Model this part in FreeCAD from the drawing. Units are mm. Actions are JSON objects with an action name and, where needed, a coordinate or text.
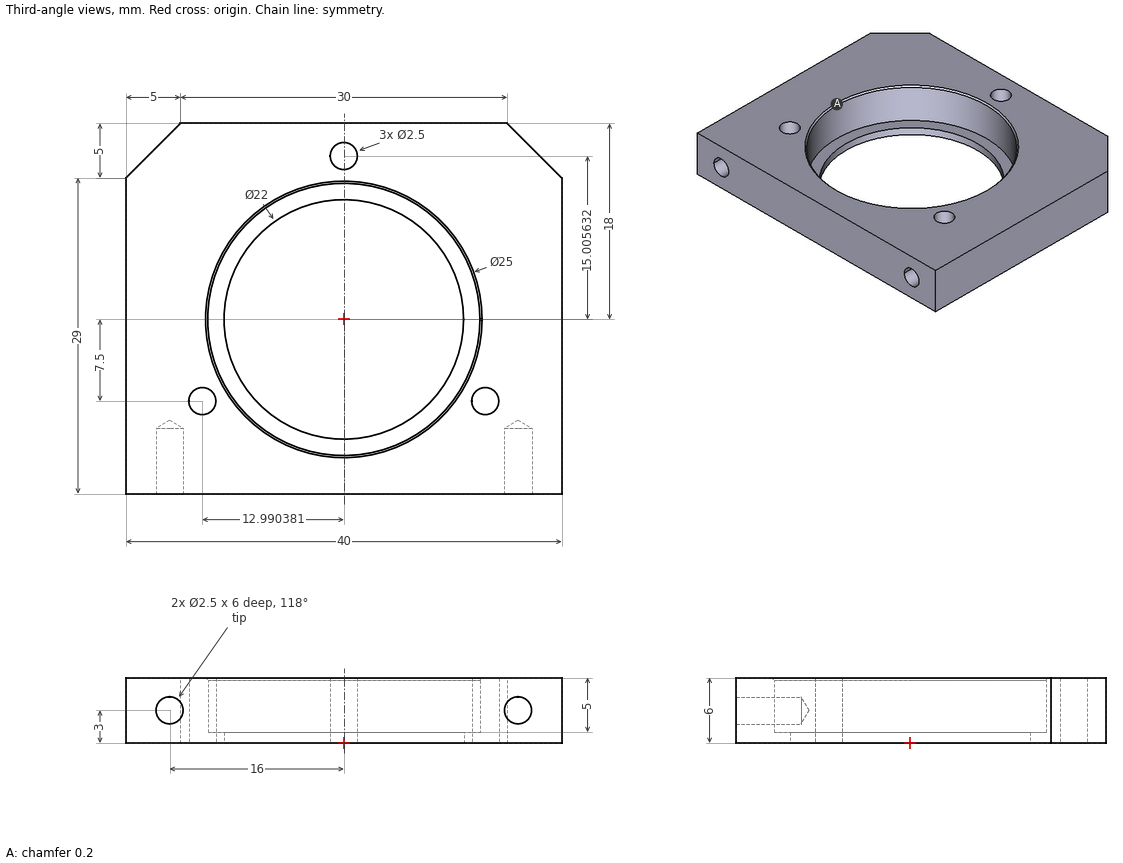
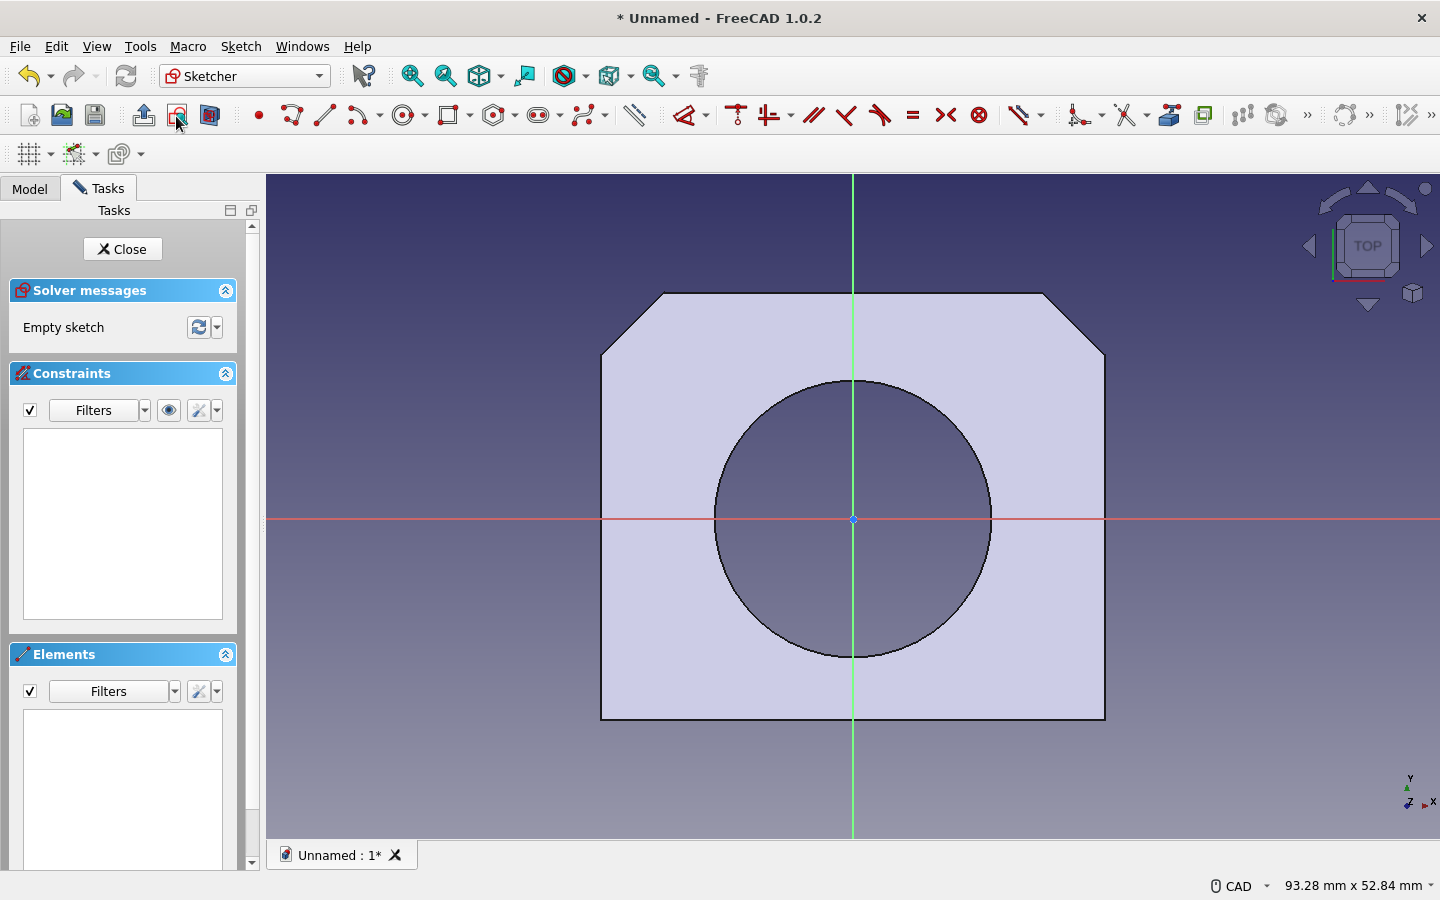
{"action": "scroll", "coordinate": [992, 545], "scroll_direction": "up", "scroll_amount": 2}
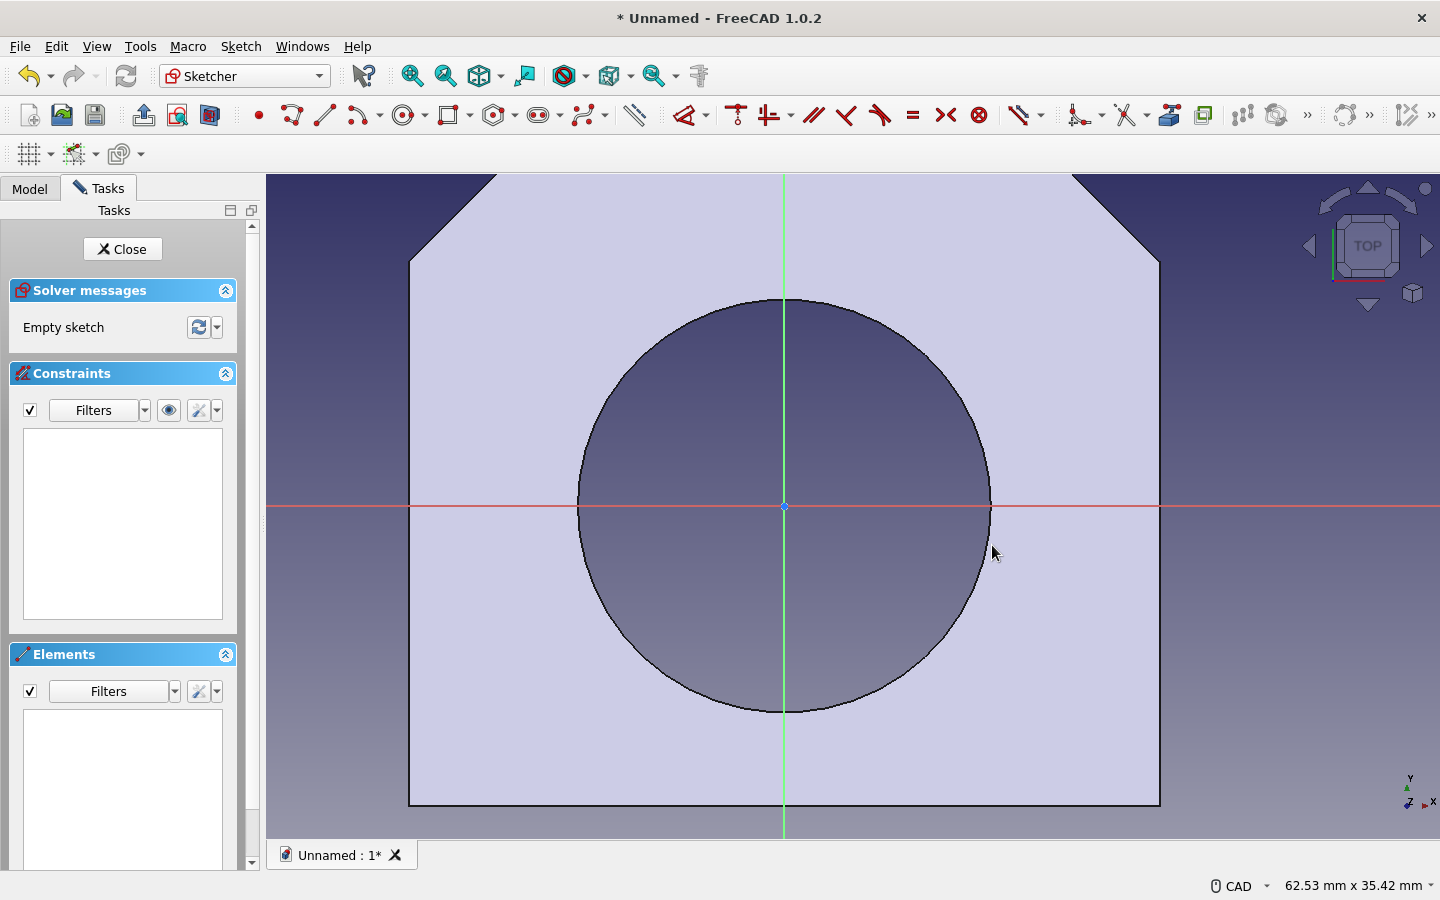
{"action": "left_click", "coordinate": [402, 116]}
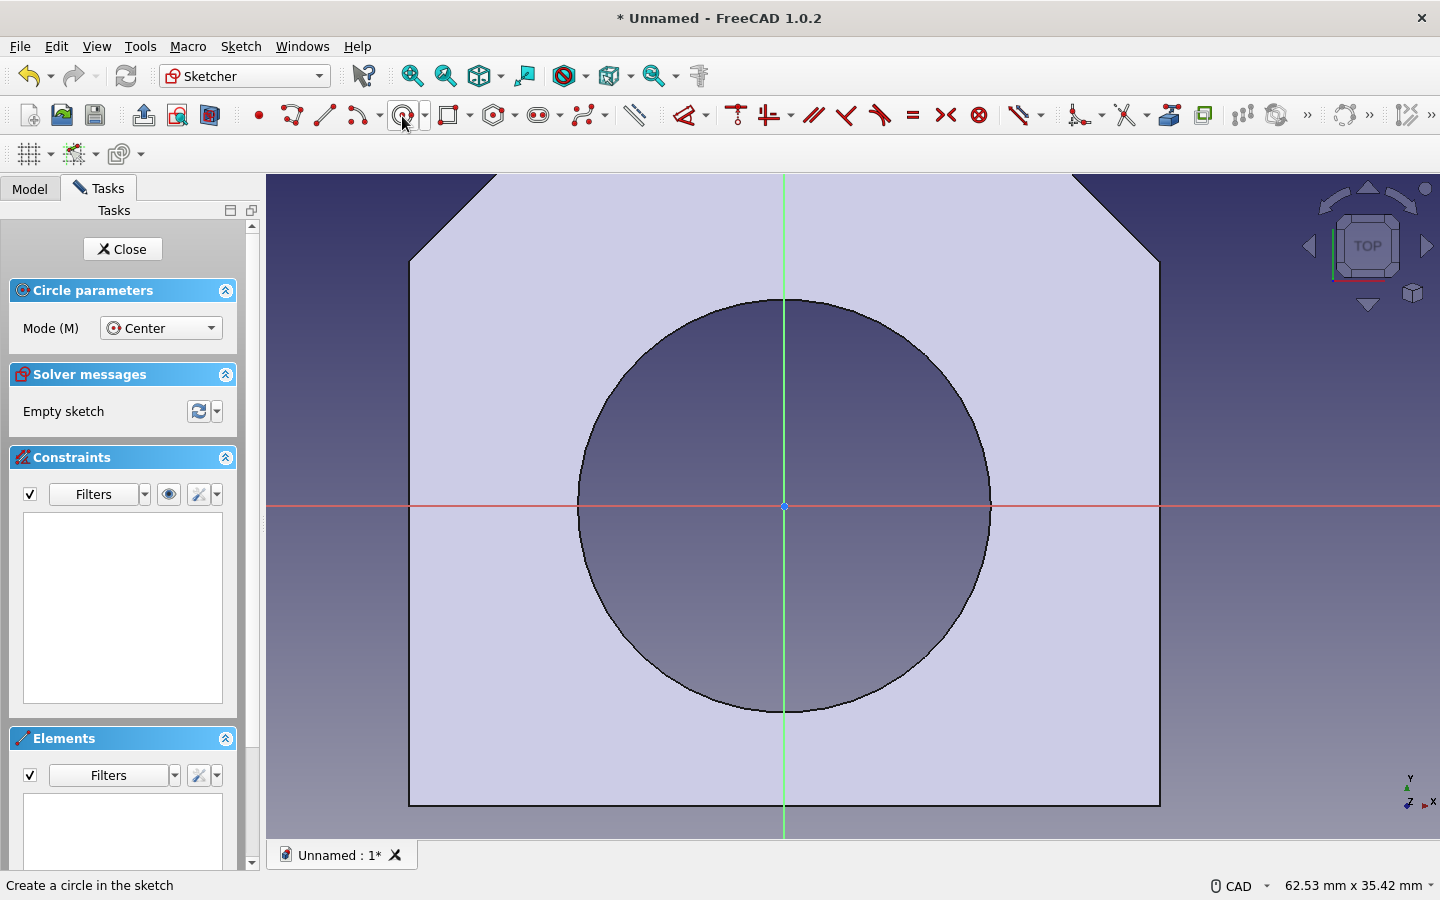
{"action": "left_click", "coordinate": [784, 506]}
{"action": "left_click", "coordinate": [950, 340]}
{"action": "key", "text": "Escape"}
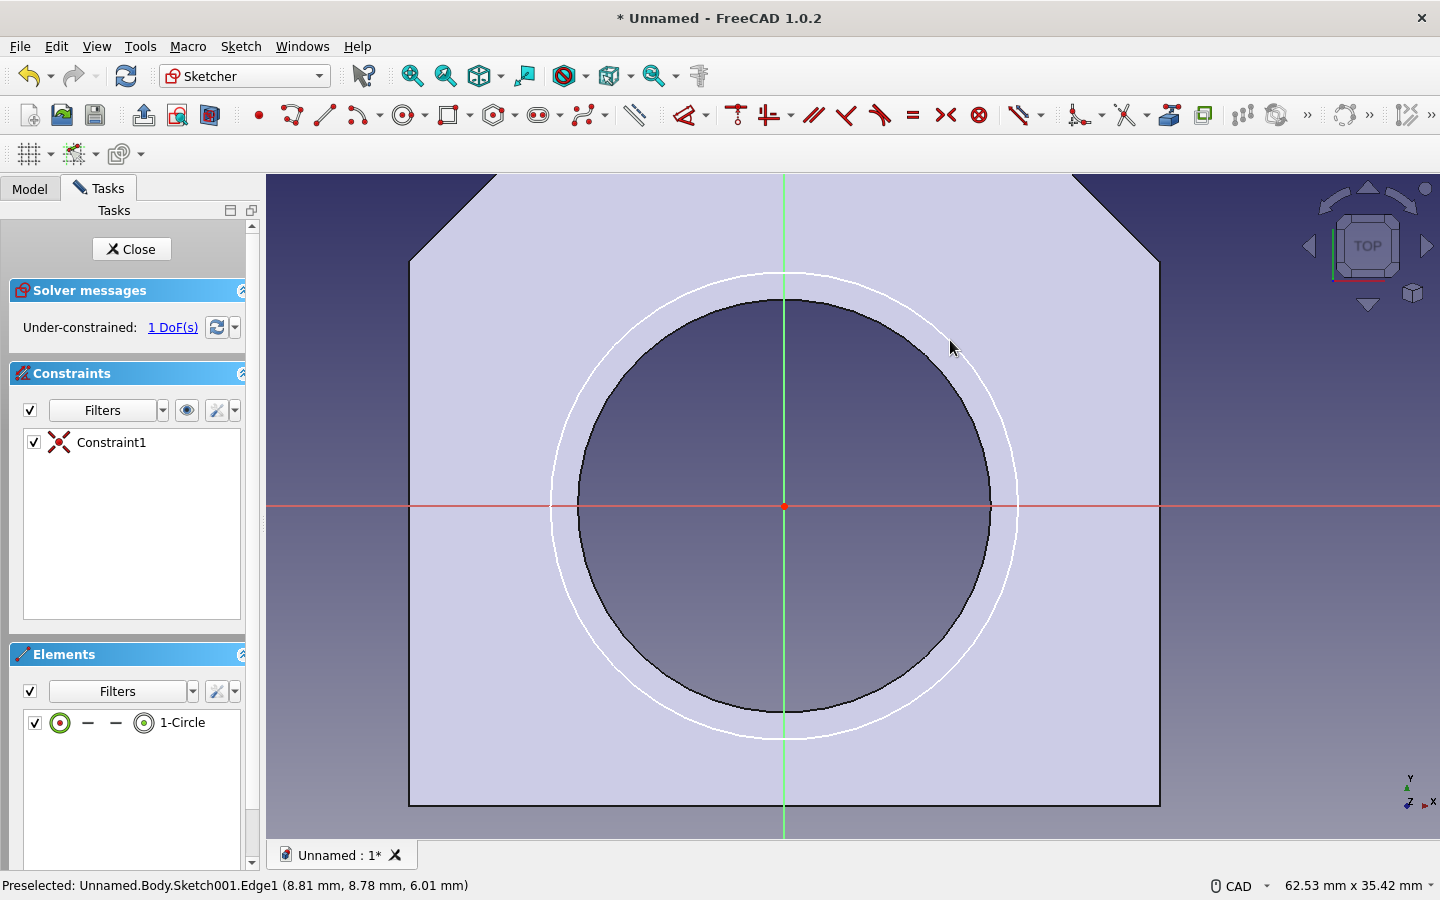
{"action": "left_click", "coordinate": [684, 116]}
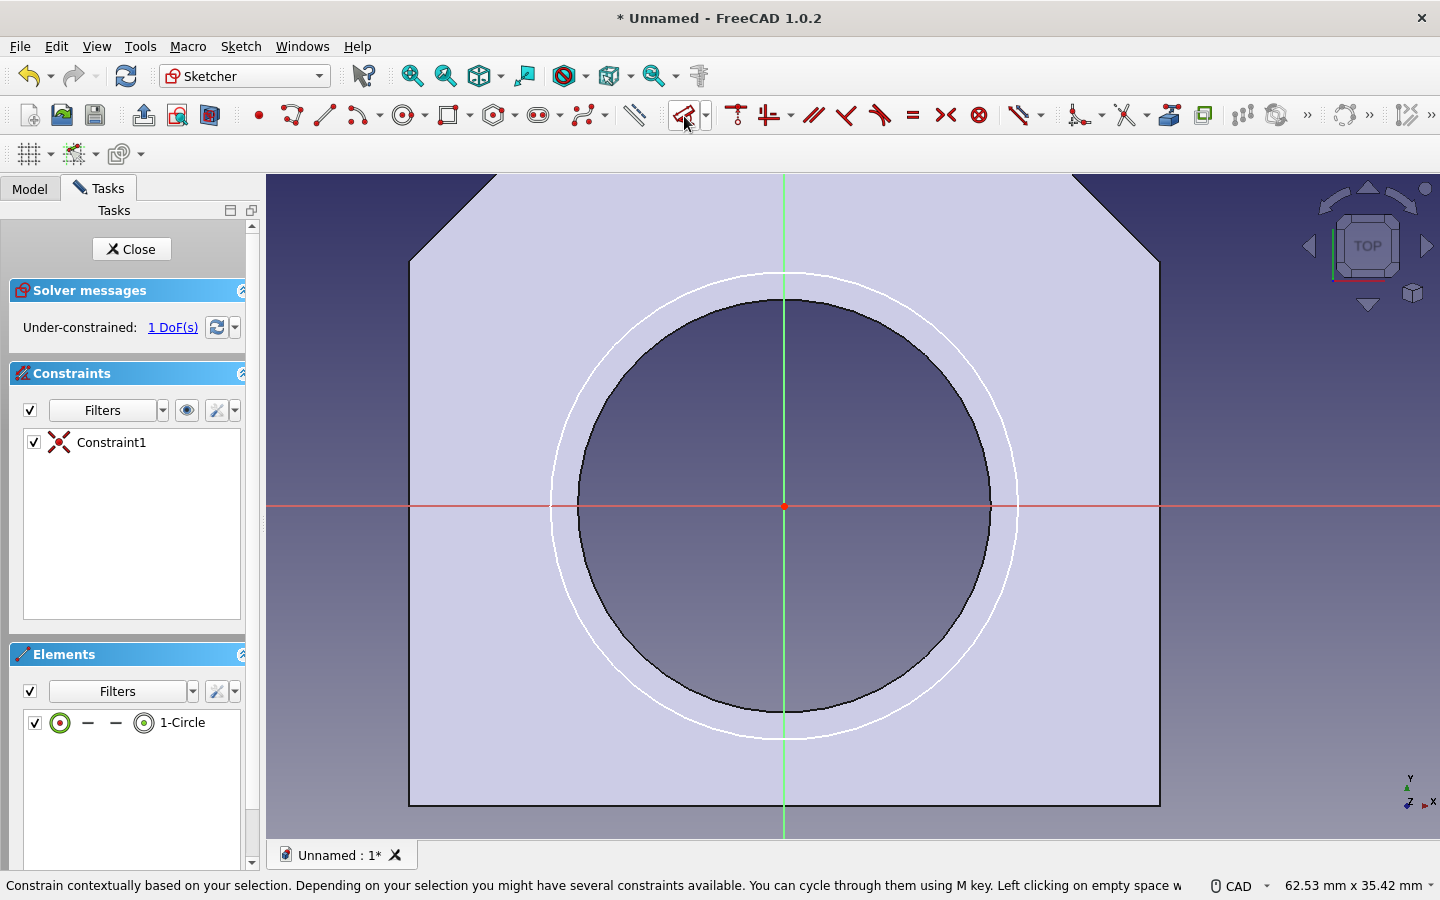
{"action": "left_click", "coordinate": [949, 340]}
{"action": "left_click", "coordinate": [972, 317]}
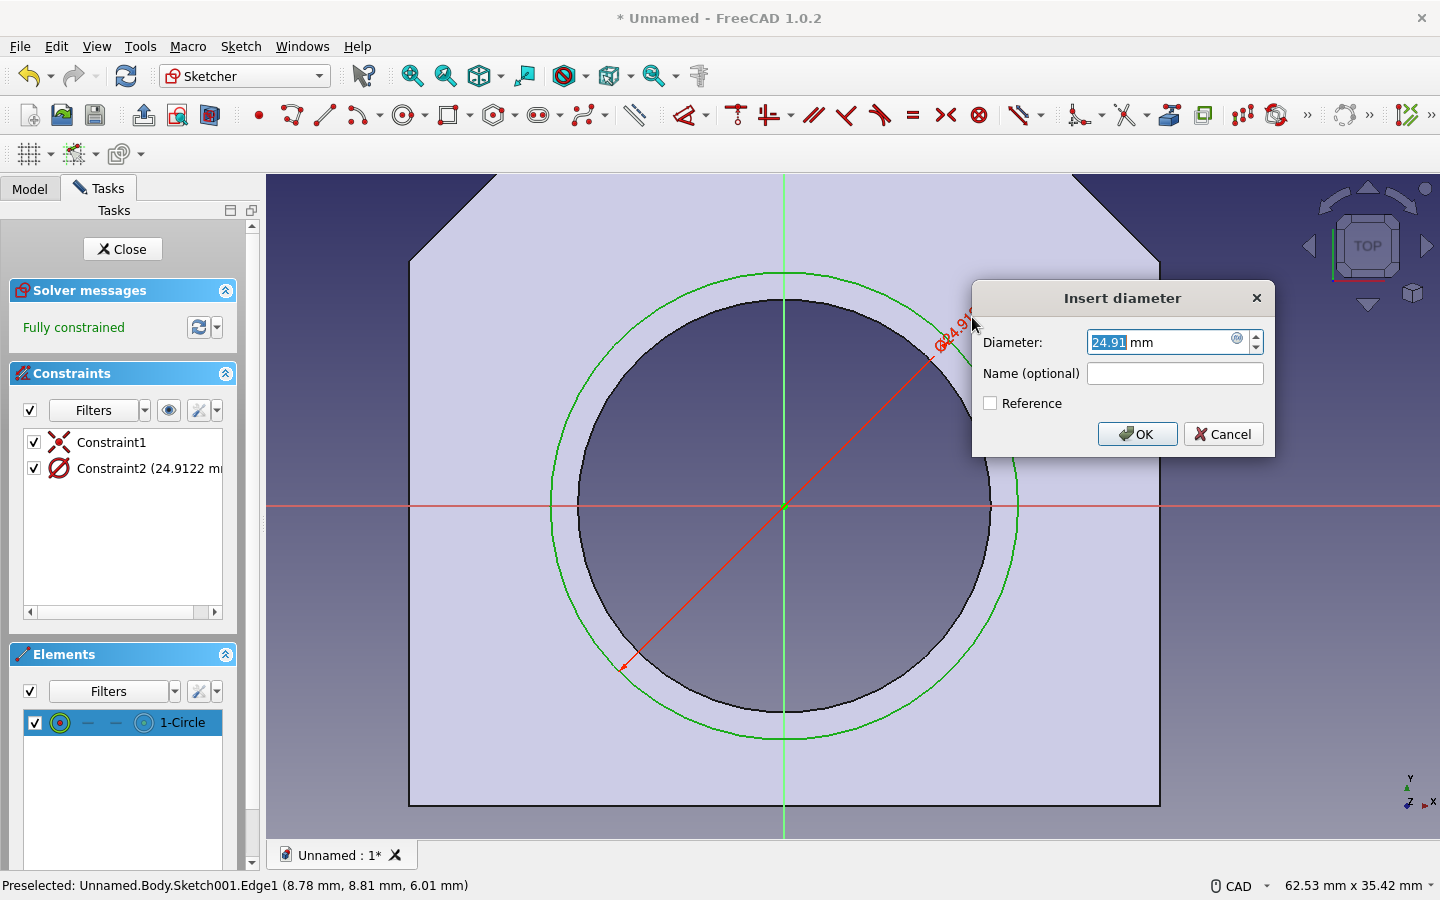
{"action": "type", "text": "25"}
{"action": "key", "text": "Return"}
{"action": "key", "text": "Escape"}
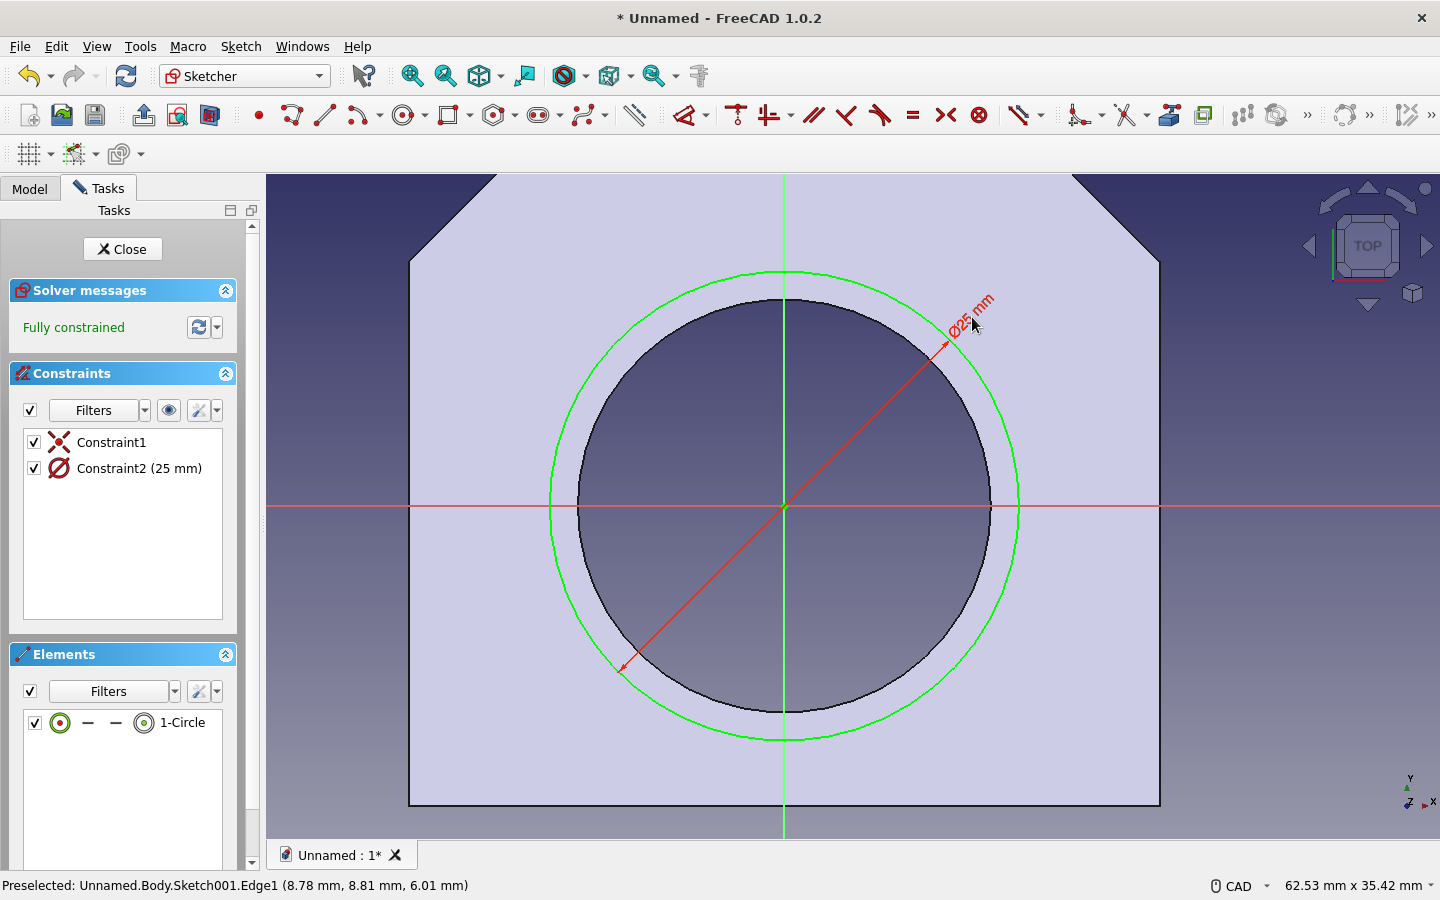
{"action": "left_click", "coordinate": [123, 249]}